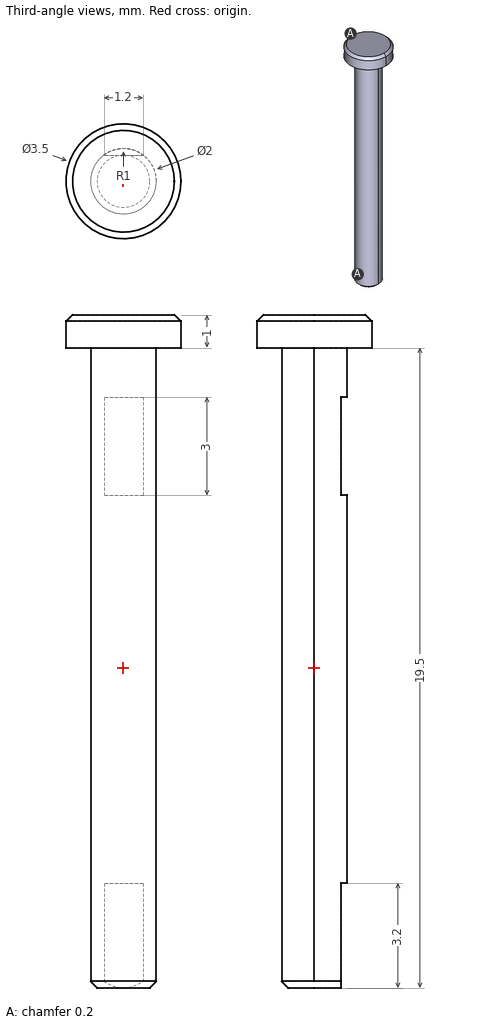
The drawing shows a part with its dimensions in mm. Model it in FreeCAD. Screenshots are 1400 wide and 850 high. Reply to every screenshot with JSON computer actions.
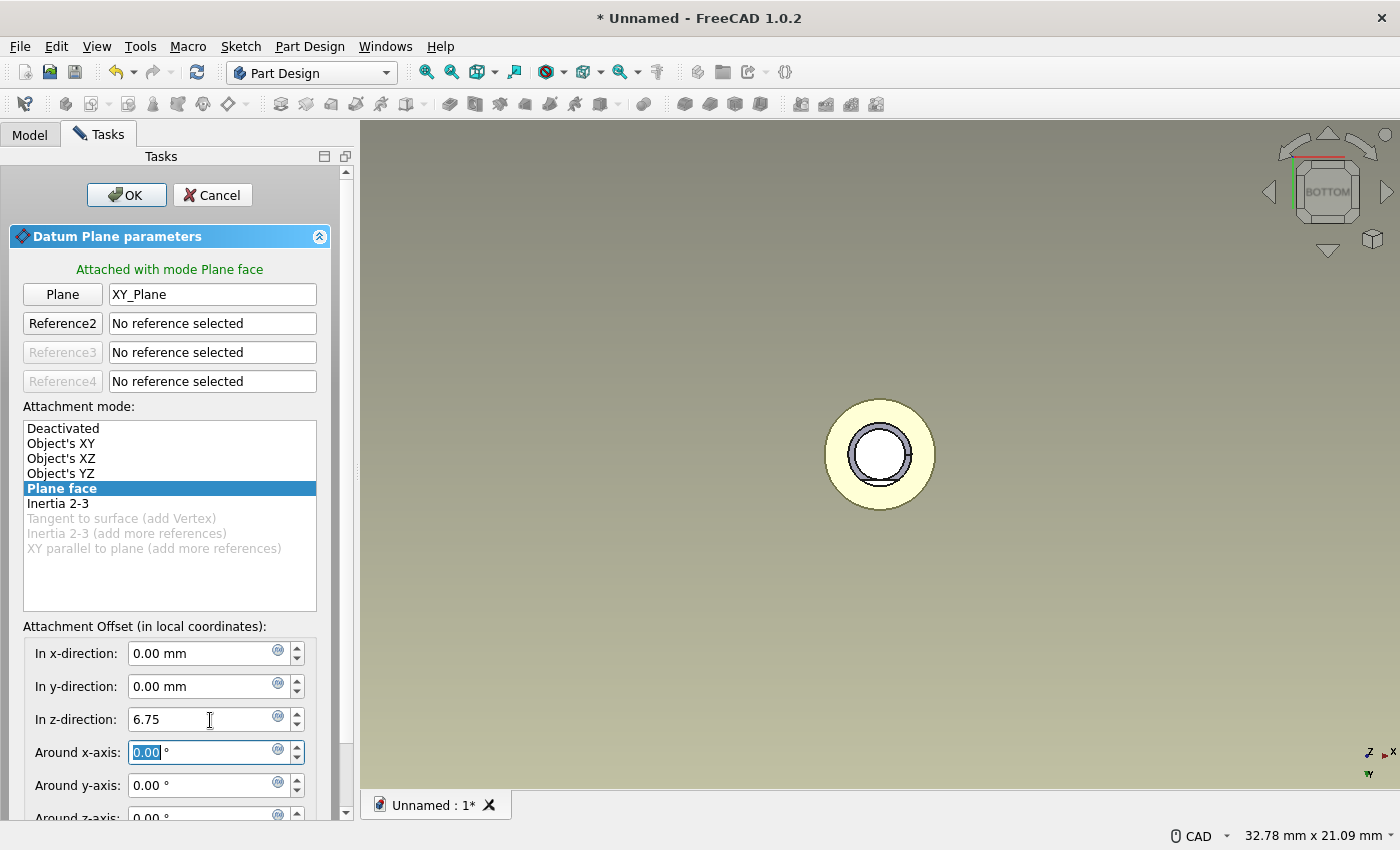
{"action": "left_click", "coordinate": [127, 195]}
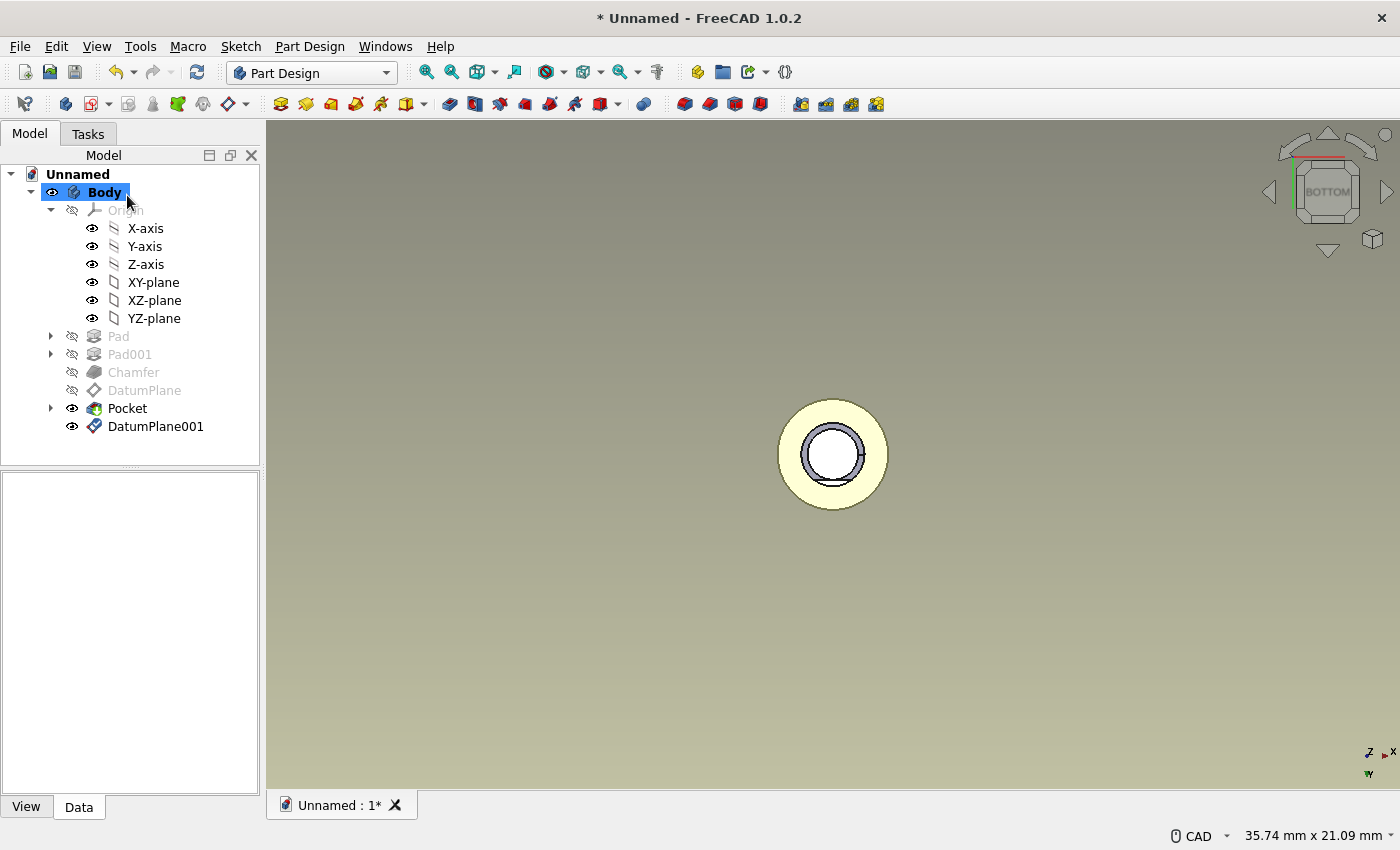
{"action": "left_click", "coordinate": [117, 426]}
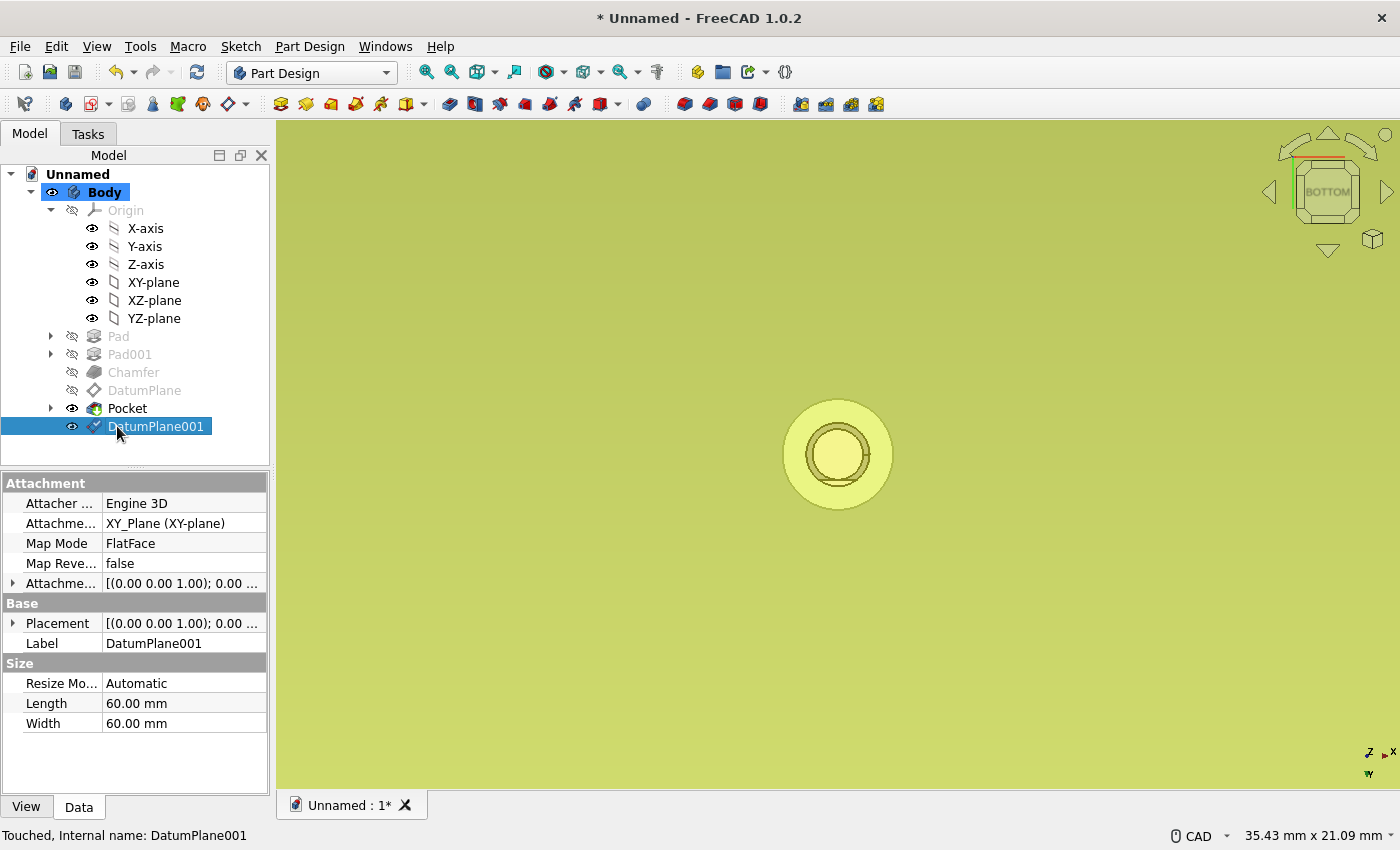
{"action": "left_click", "coordinate": [90, 104]}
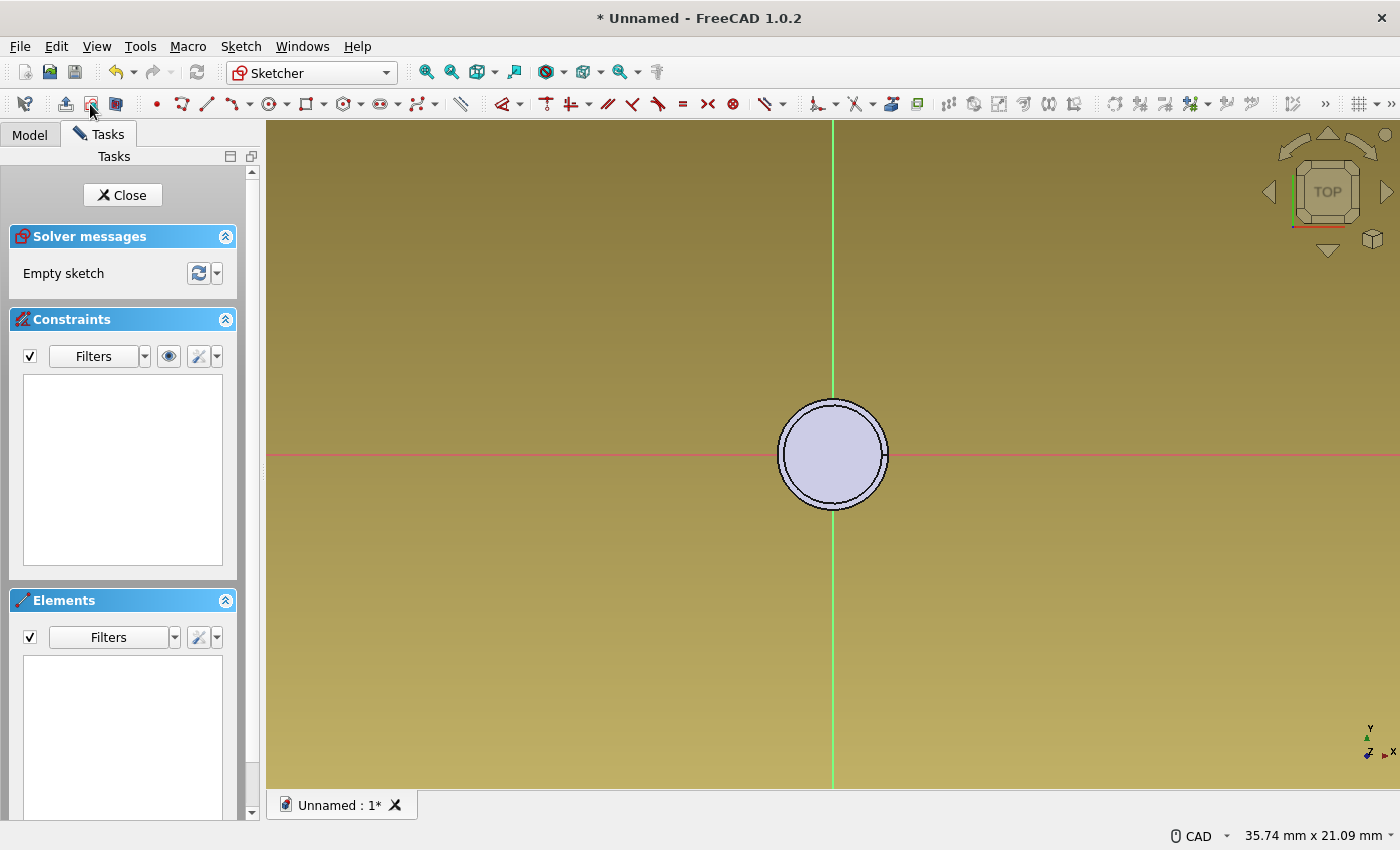
{"action": "key", "text": "q s"}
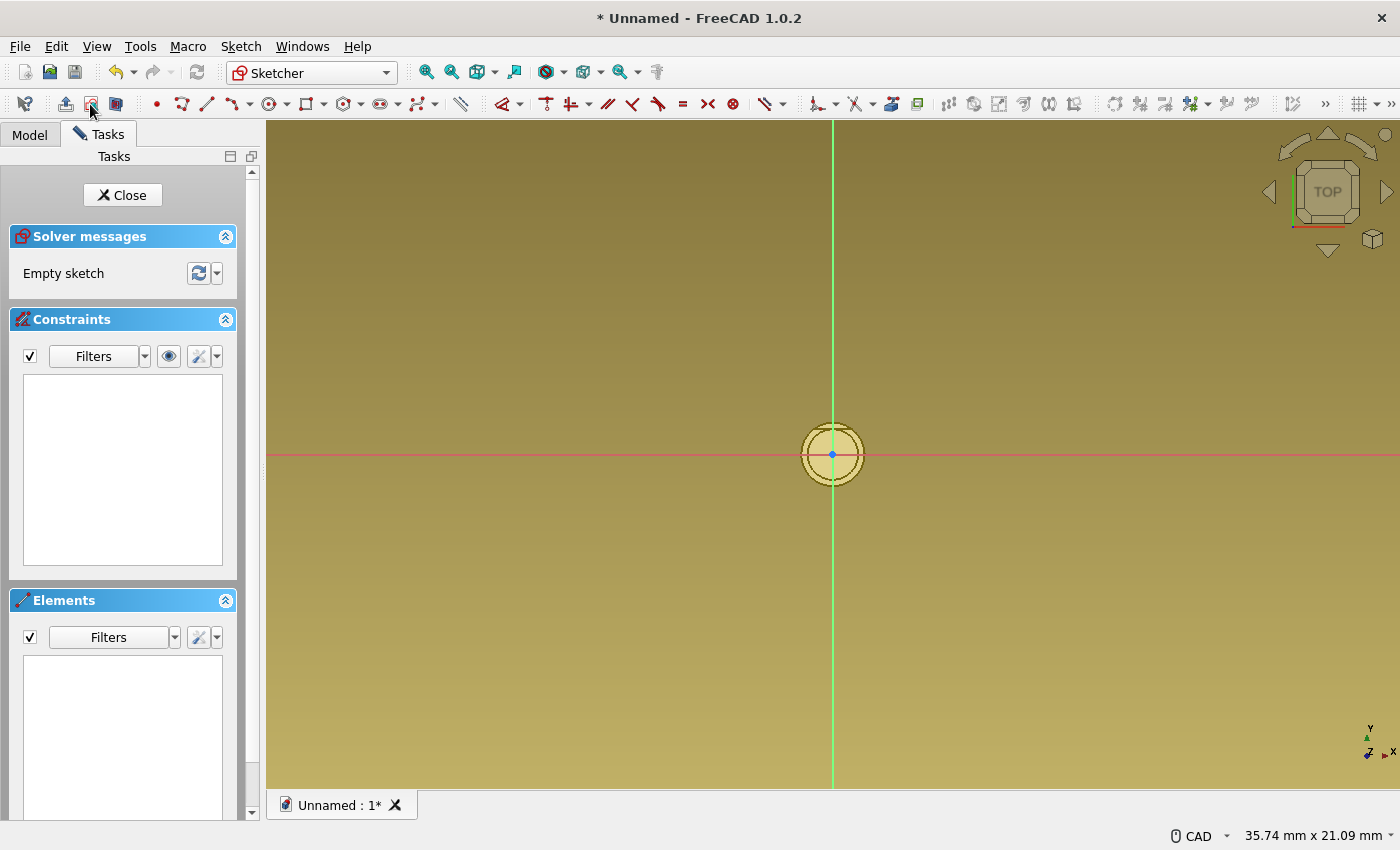
{"action": "scroll", "coordinate": [838, 437], "scroll_direction": "up", "scroll_amount": 13}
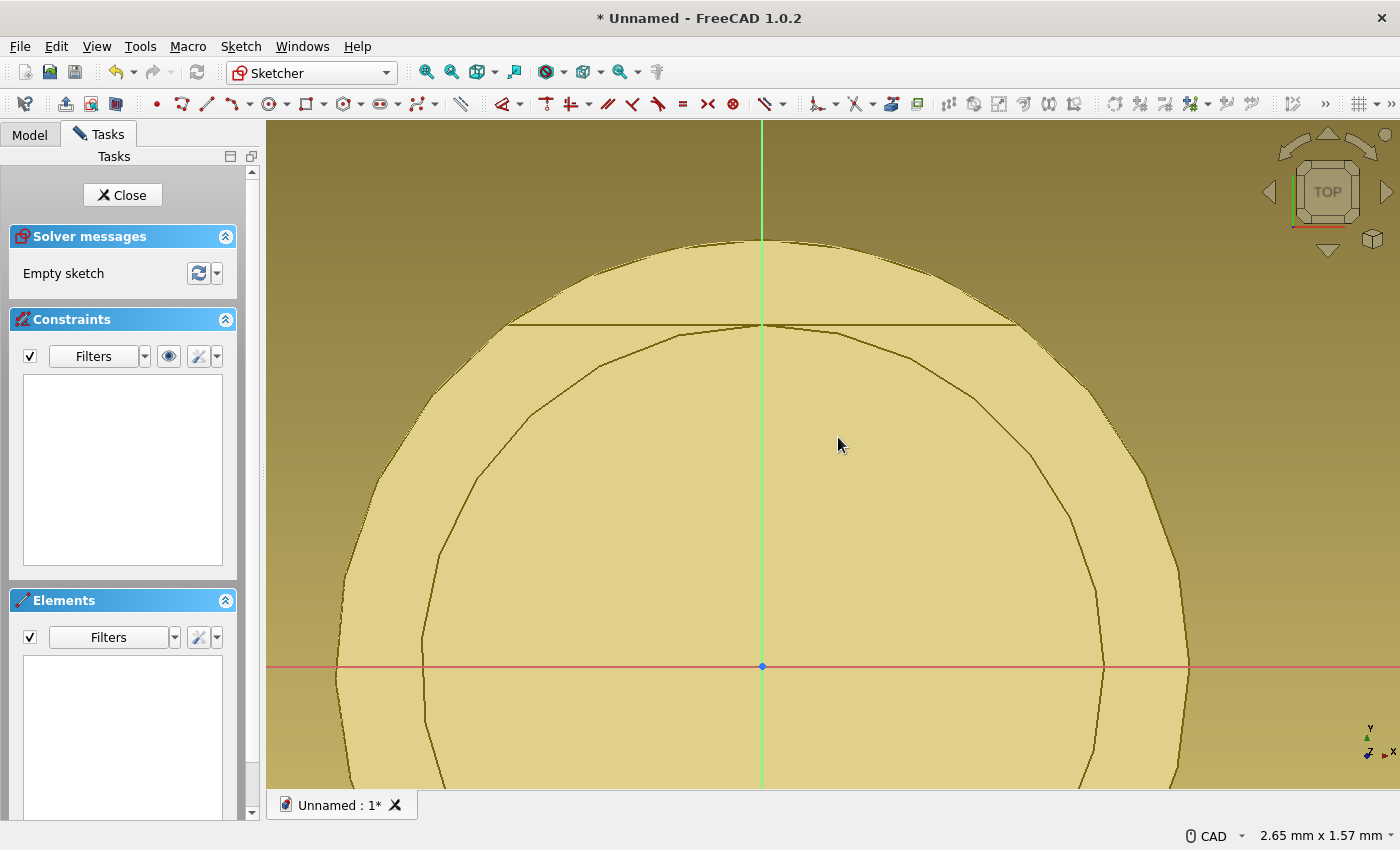
{"action": "left_click", "coordinate": [207, 104]}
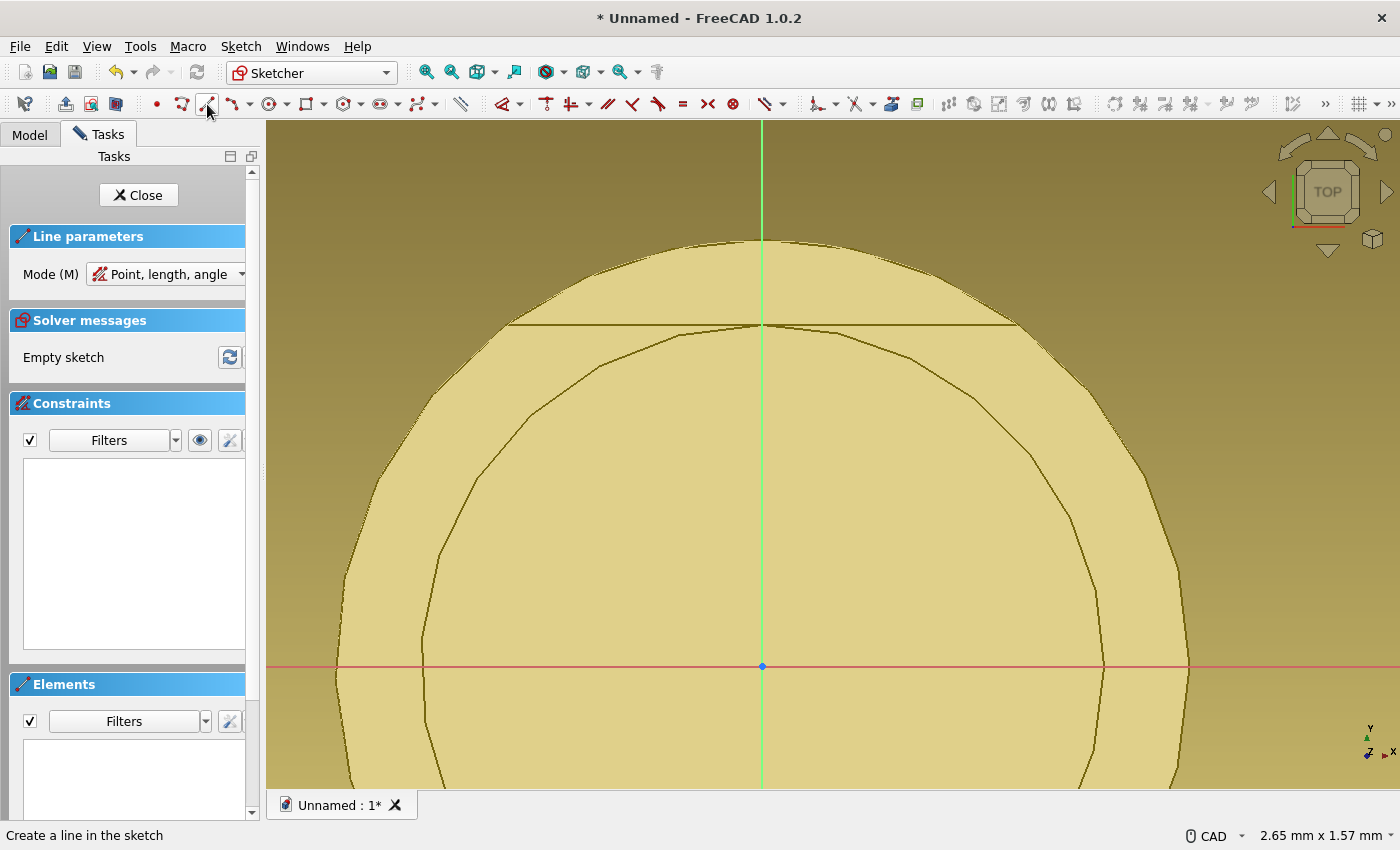
{"action": "left_click", "coordinate": [1019, 325]}
{"action": "left_click", "coordinate": [506, 325]}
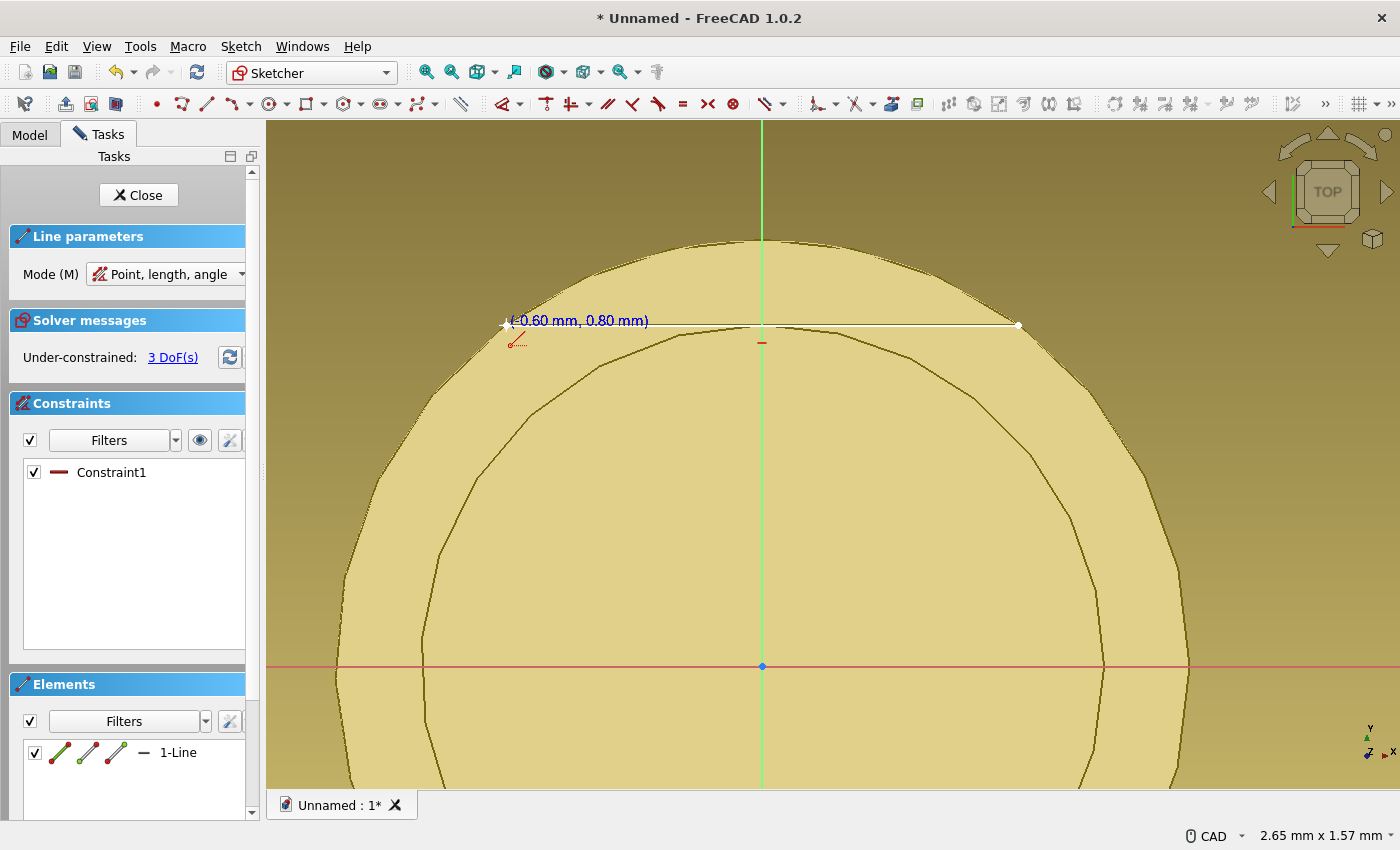
{"action": "left_click", "coordinate": [232, 104]}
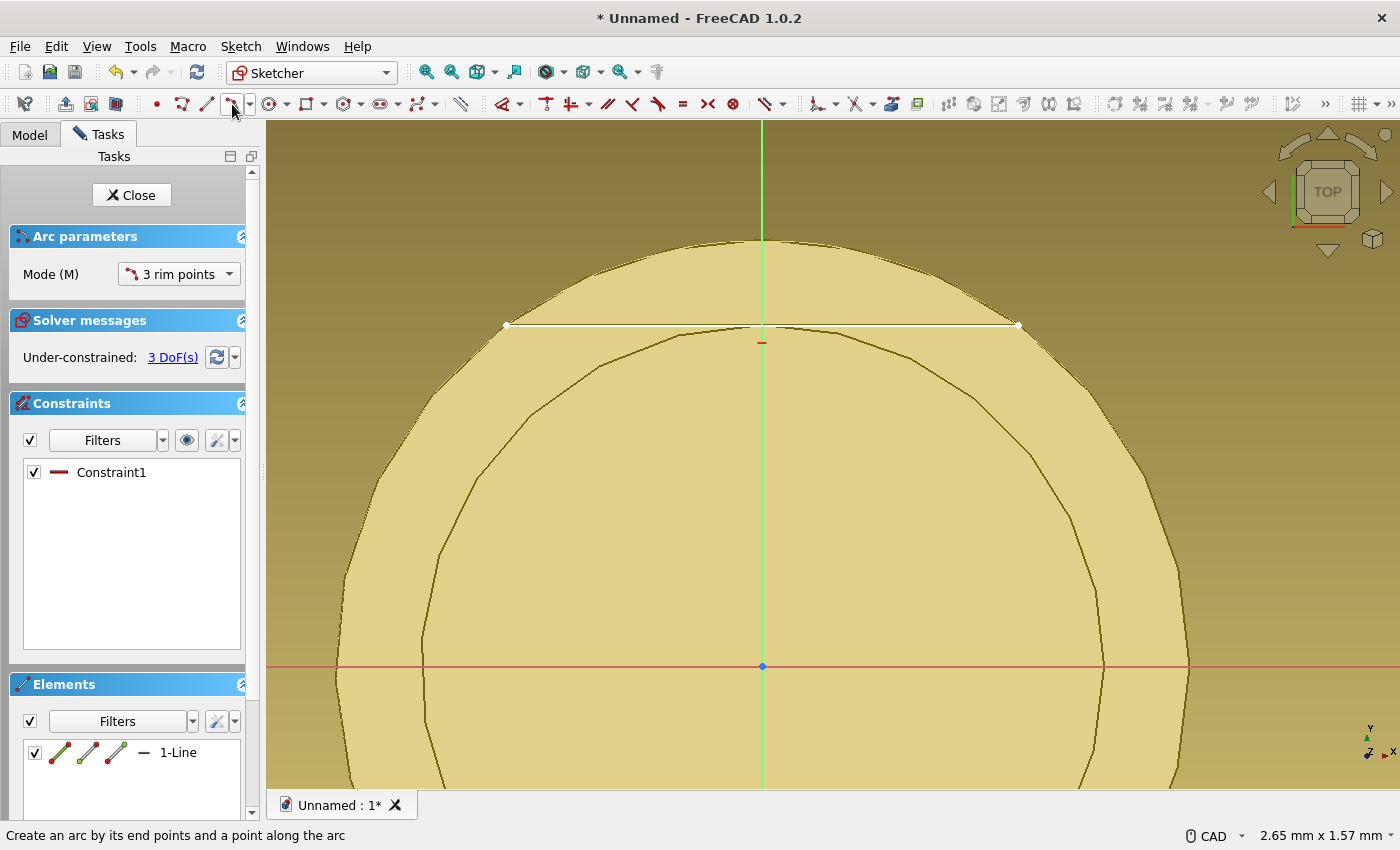
{"action": "left_click", "coordinate": [506, 326]}
{"action": "left_click", "coordinate": [1019, 326]}
{"action": "left_click", "coordinate": [817, 243]}
{"action": "key", "text": "Escape"}